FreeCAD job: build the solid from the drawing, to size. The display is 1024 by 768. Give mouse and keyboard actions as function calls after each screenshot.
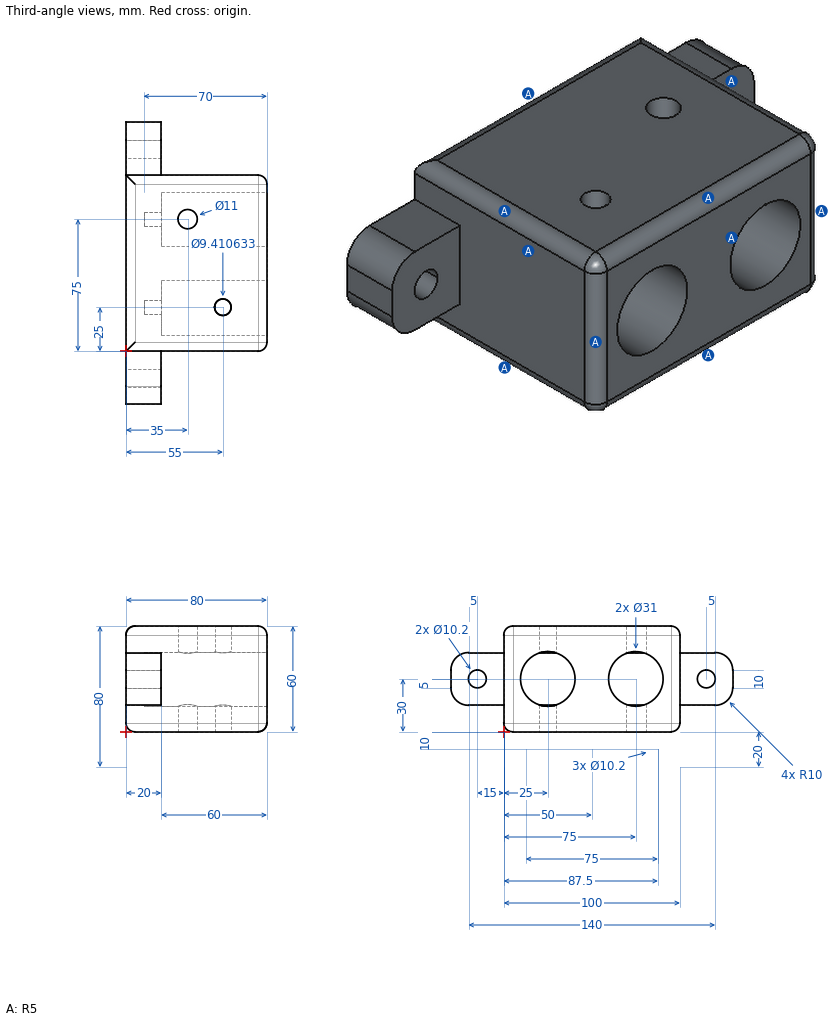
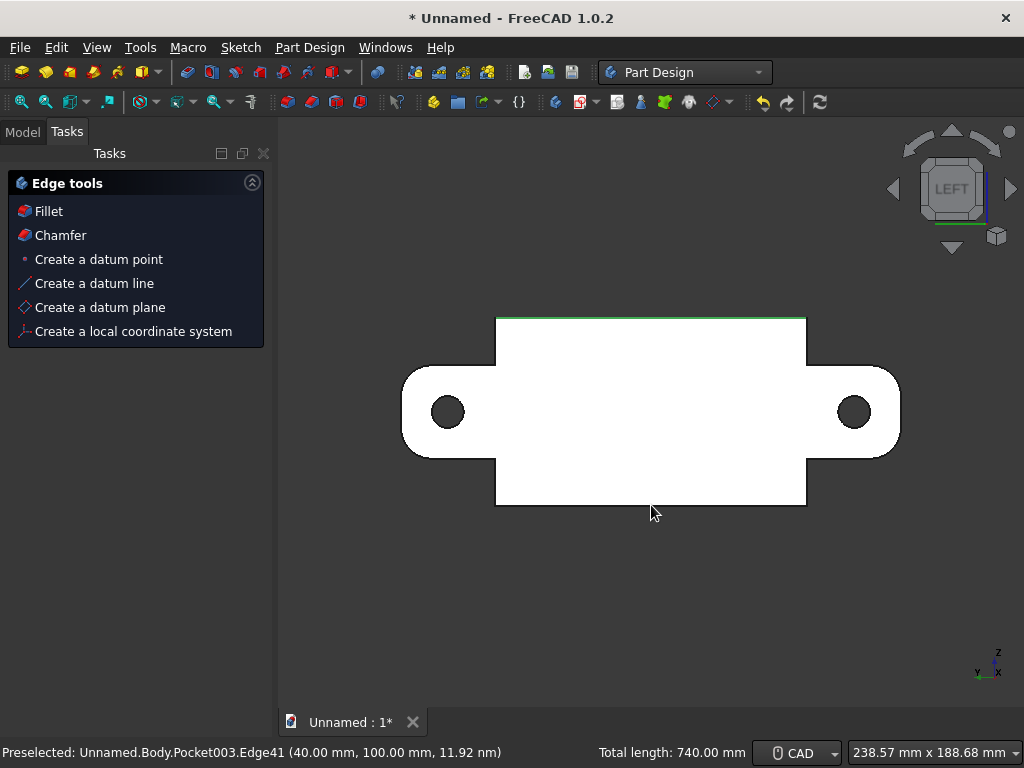
key(v)
key(3)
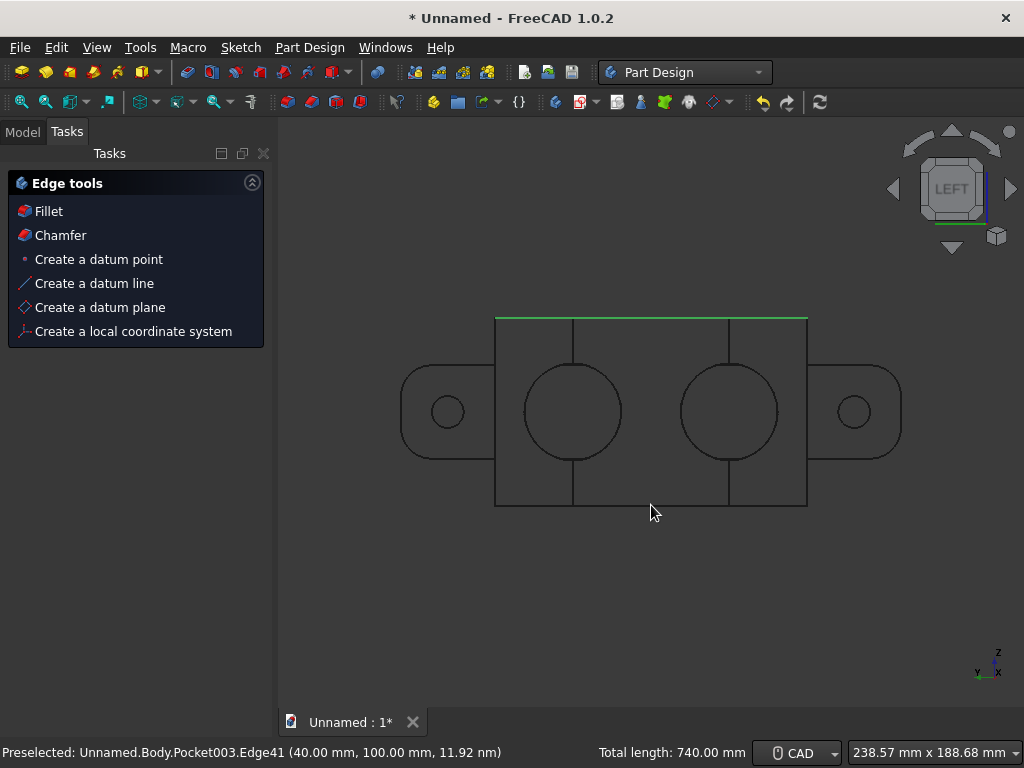
key(0)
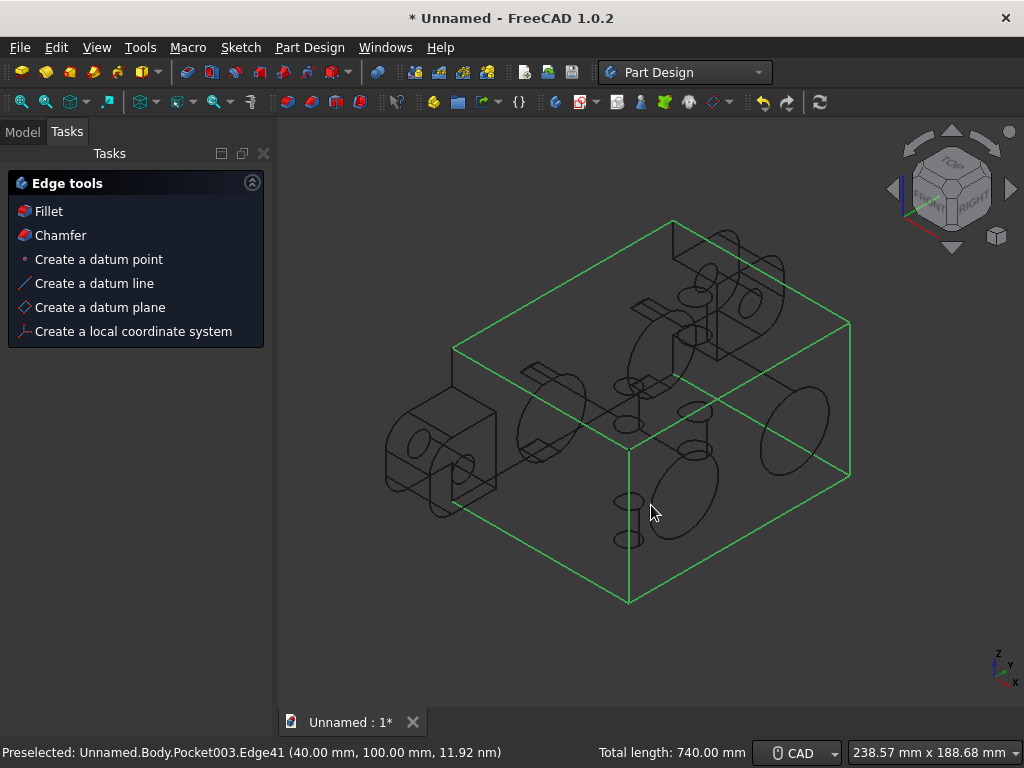
click(563, 437, ctrl)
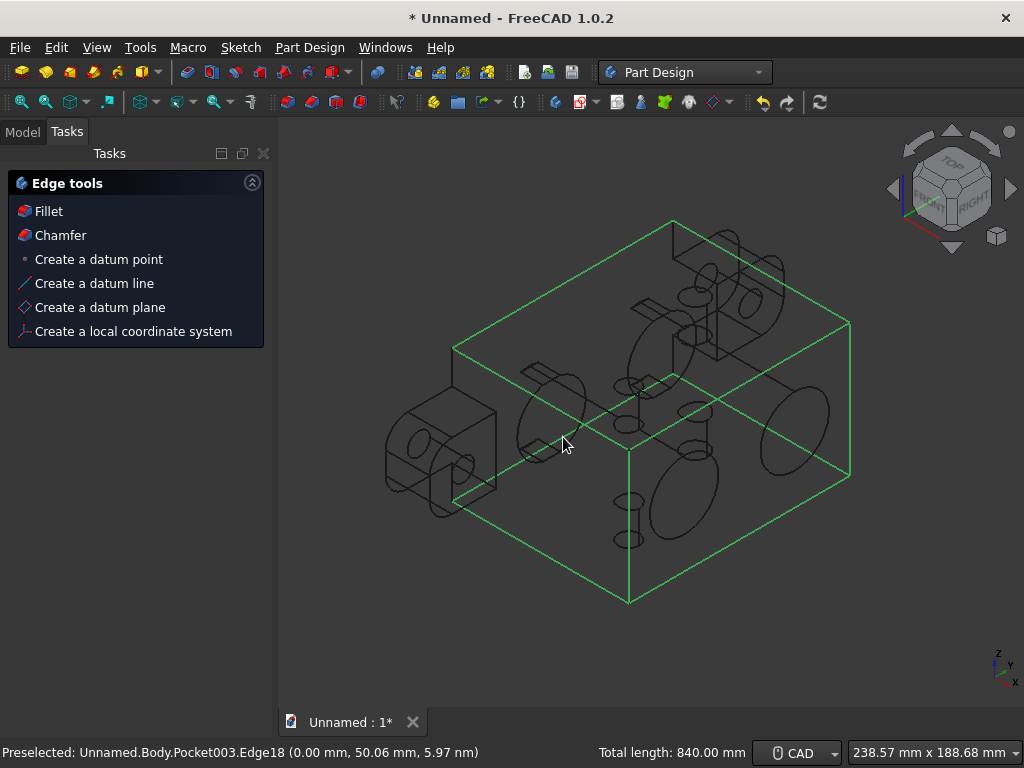
key(v)
key(1)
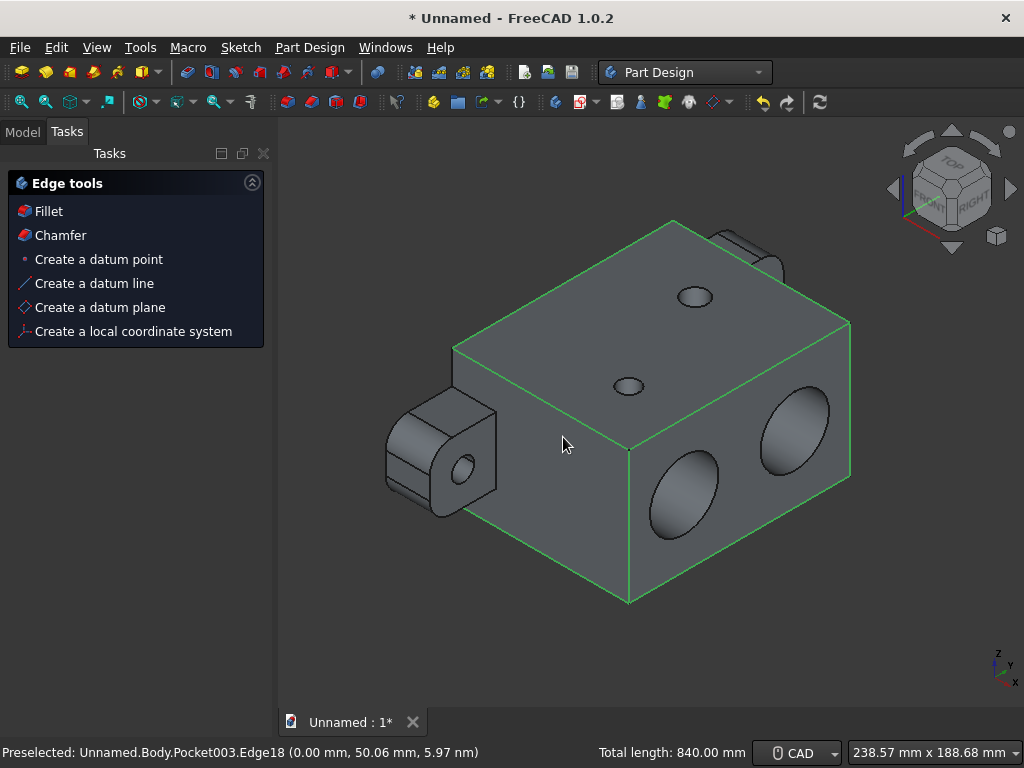
click(288, 102)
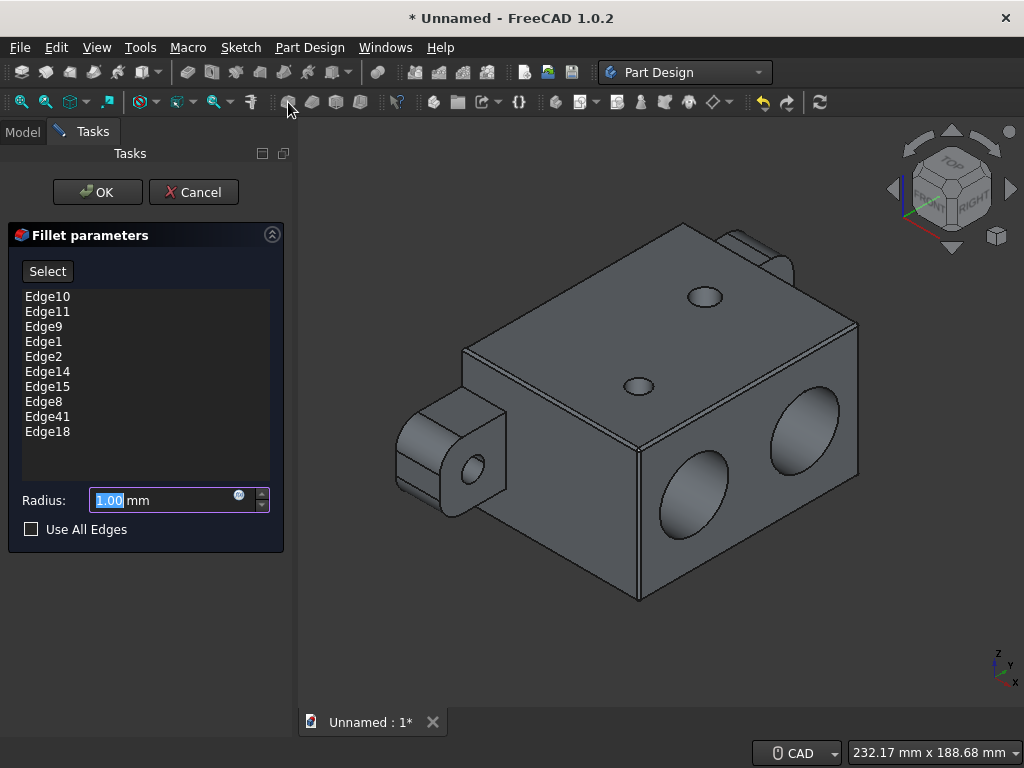
text(5)
key(Tab)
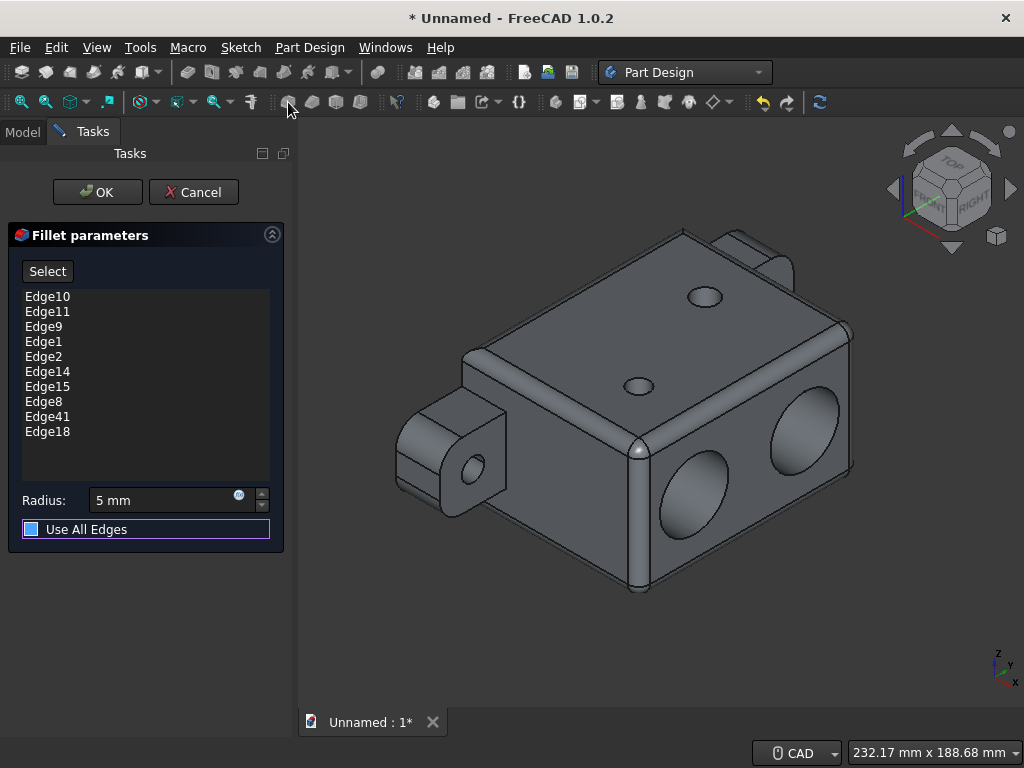
click(98, 192)